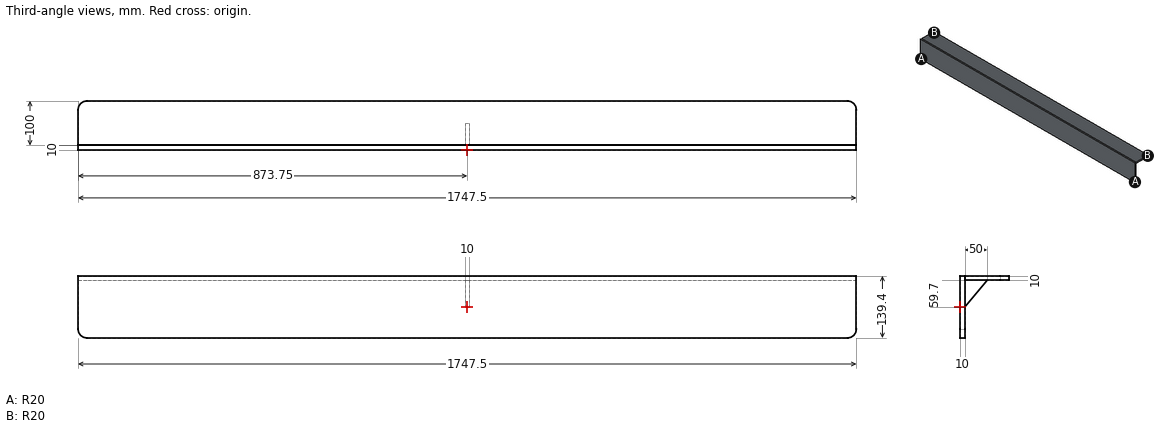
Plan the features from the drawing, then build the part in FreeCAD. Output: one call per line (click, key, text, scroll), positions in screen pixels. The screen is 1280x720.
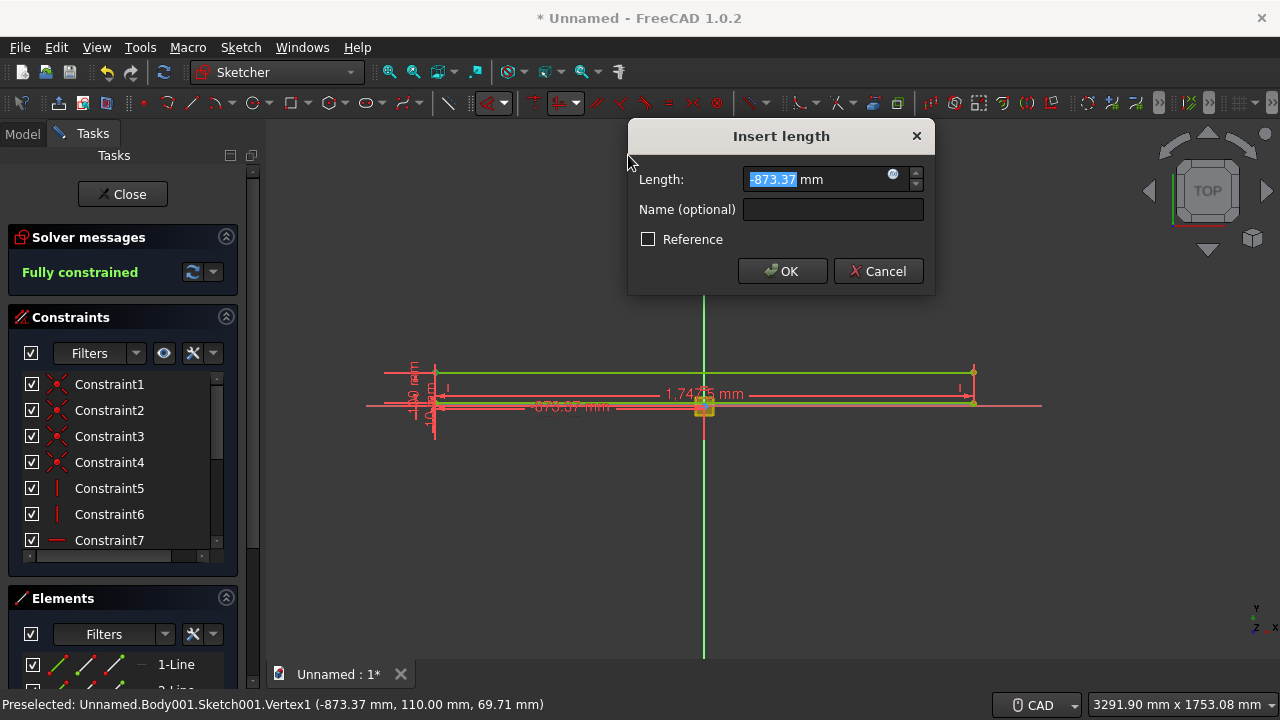
text(-873.75)
key(Return)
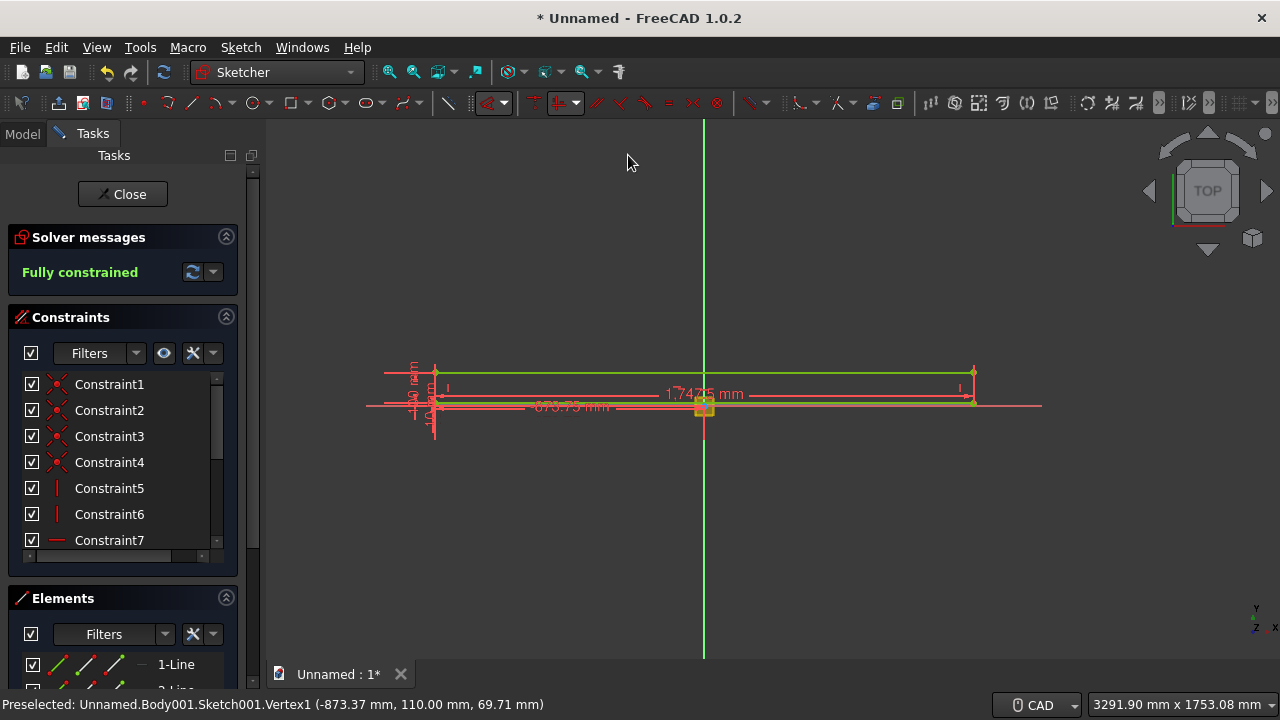
click(123, 194)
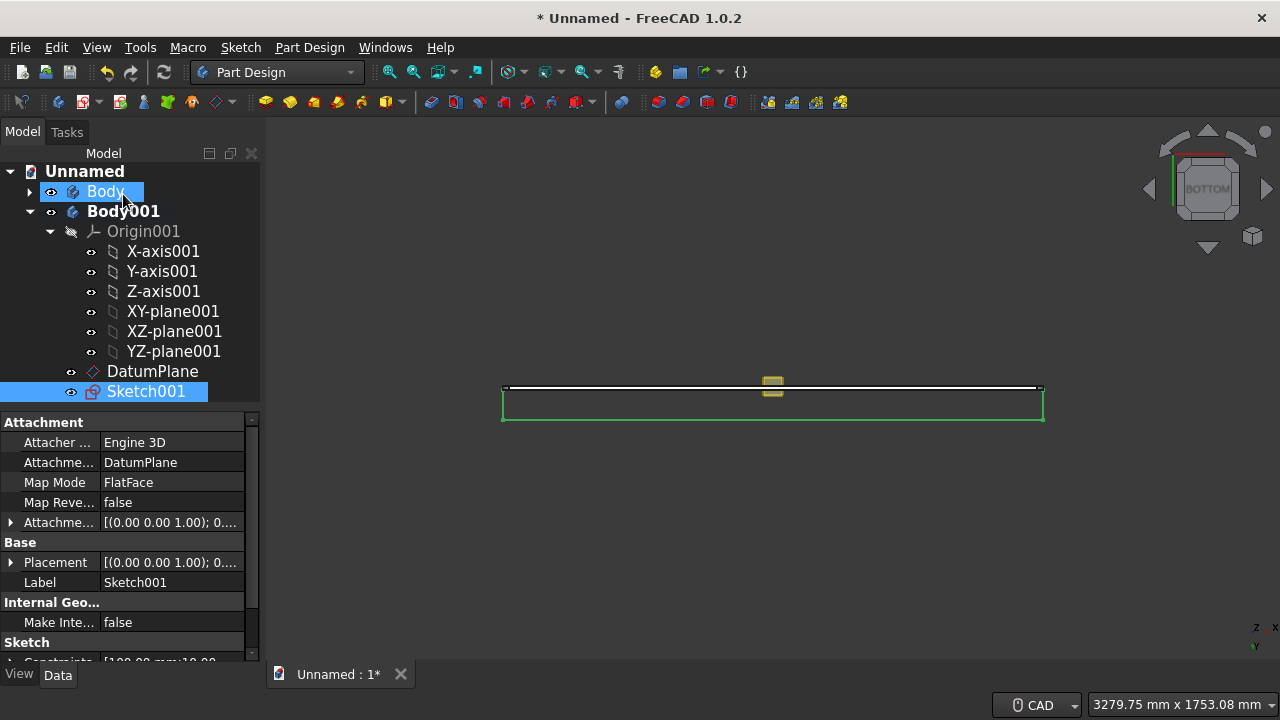
click(266, 102)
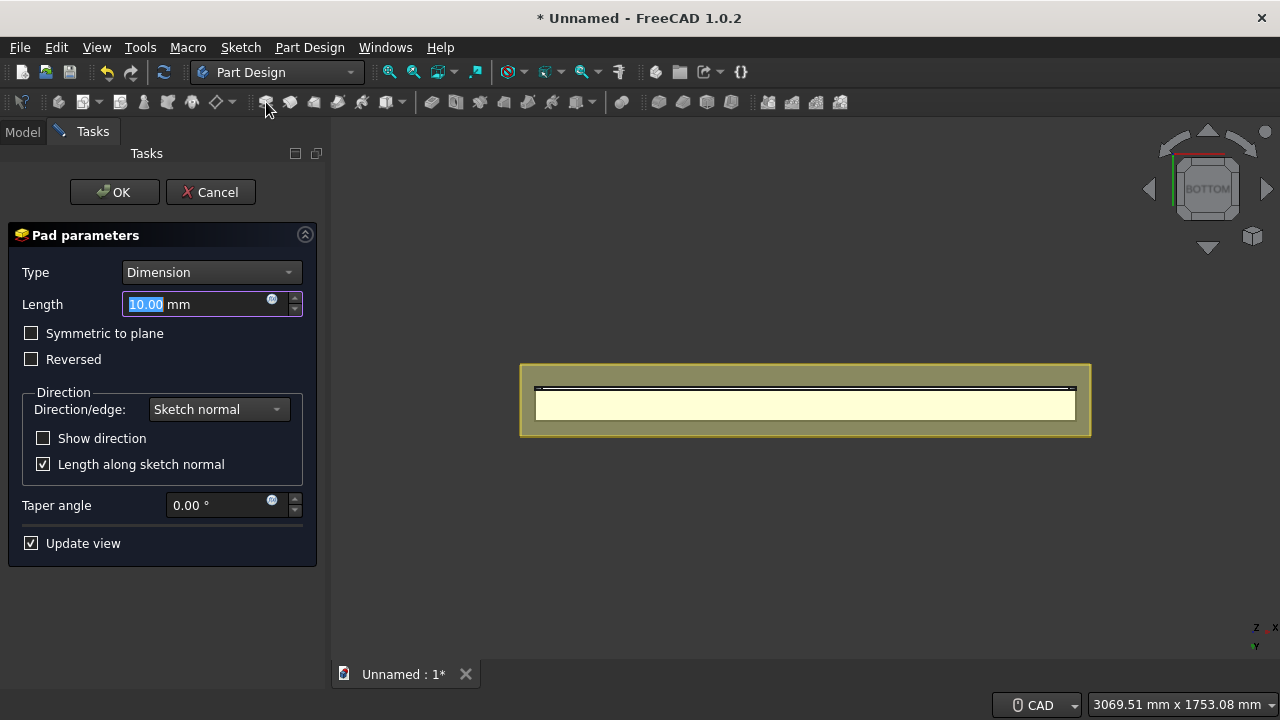
text(10)
key(Tab)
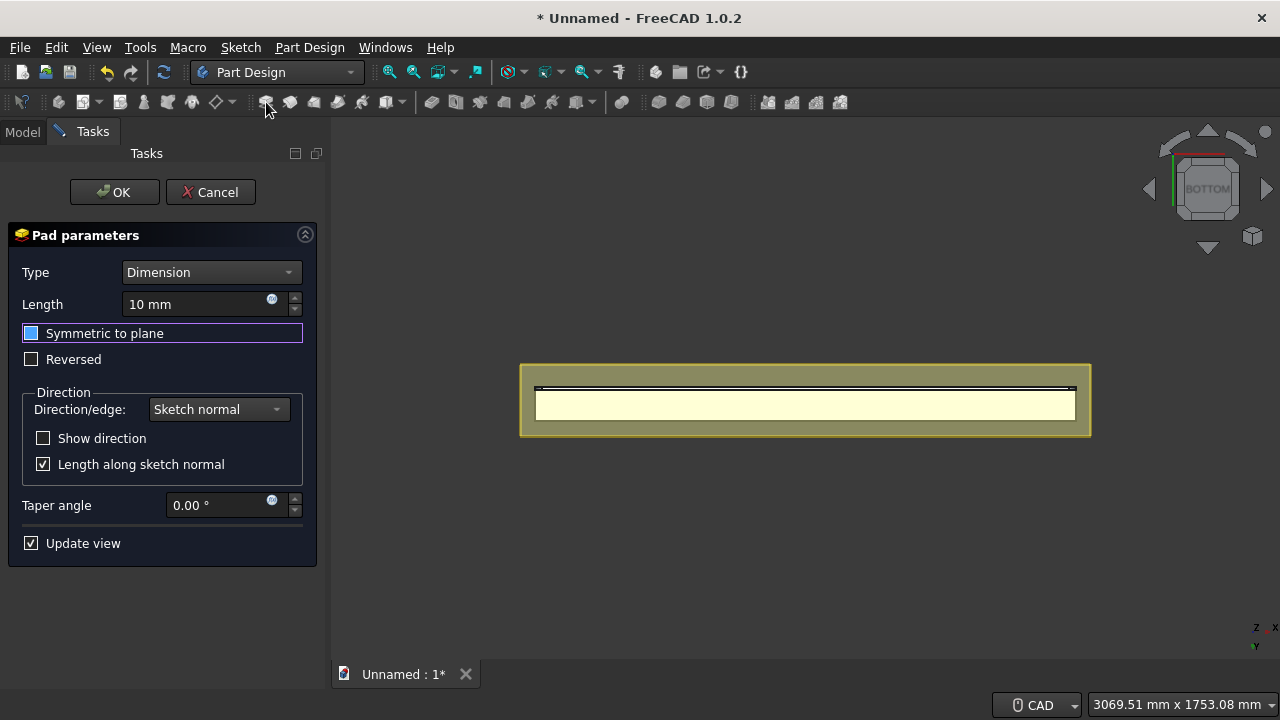
click(30, 359)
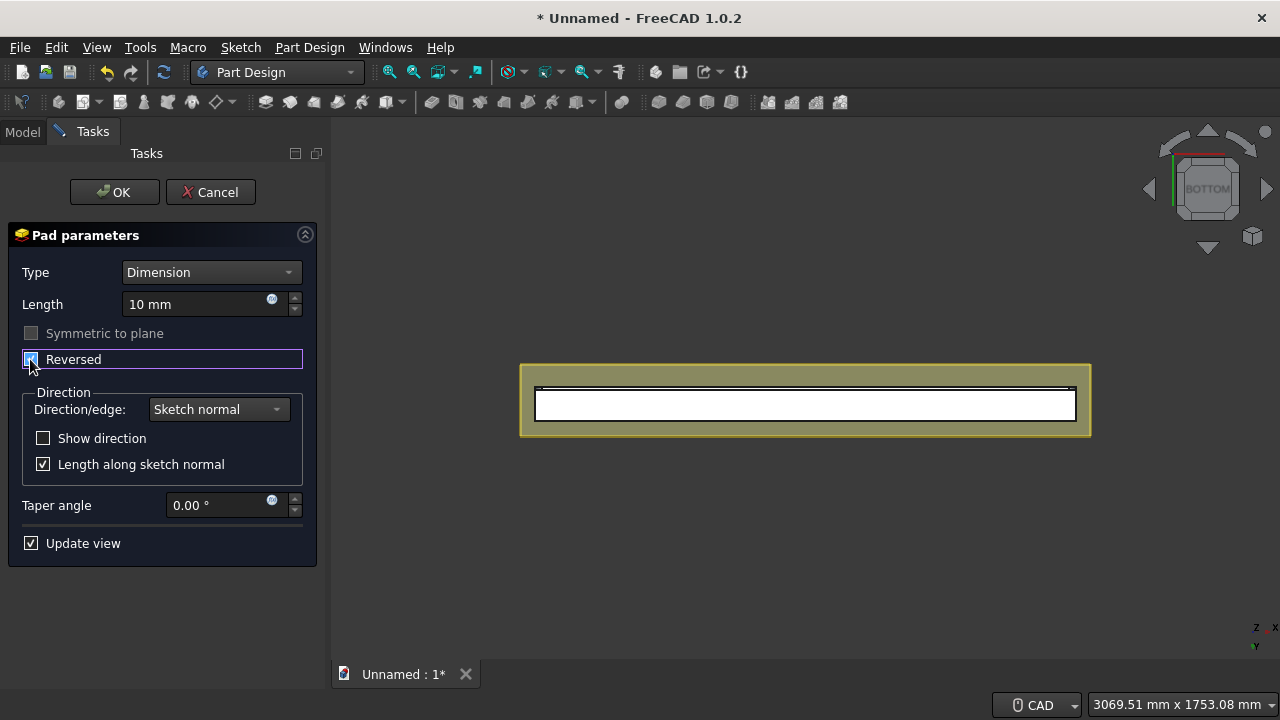
click(115, 192)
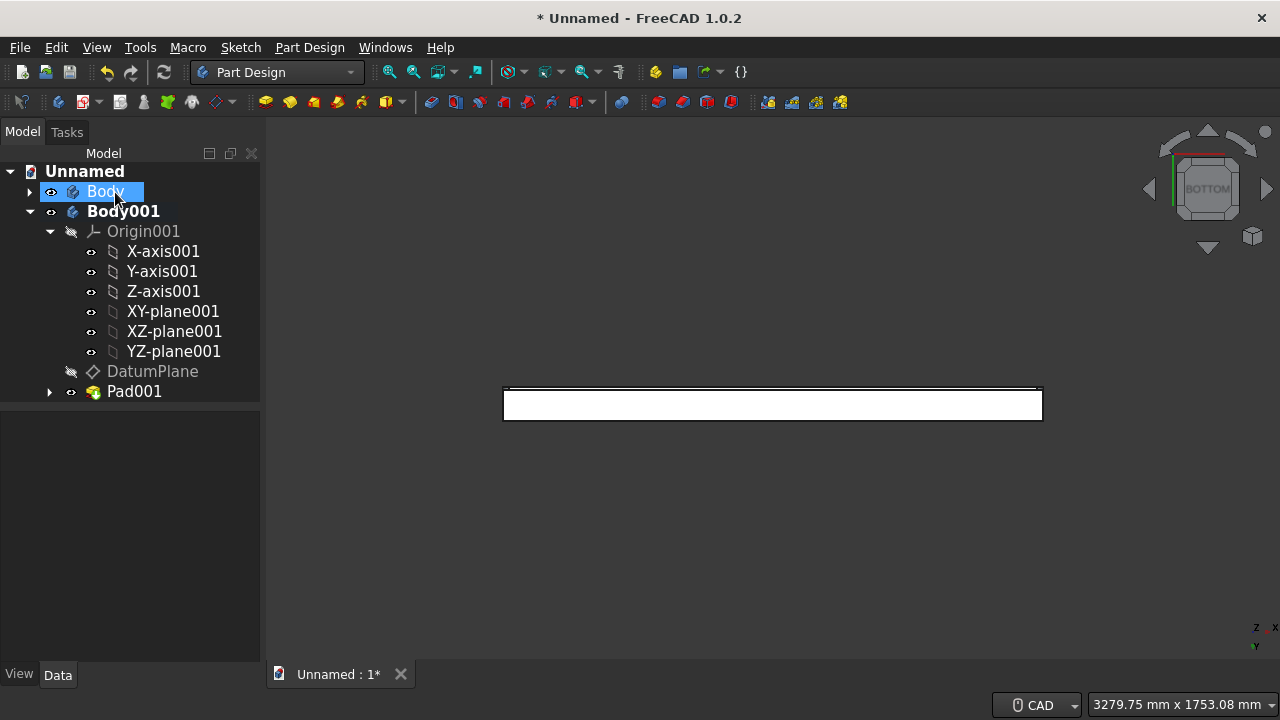
scroll(503, 420, up, 13)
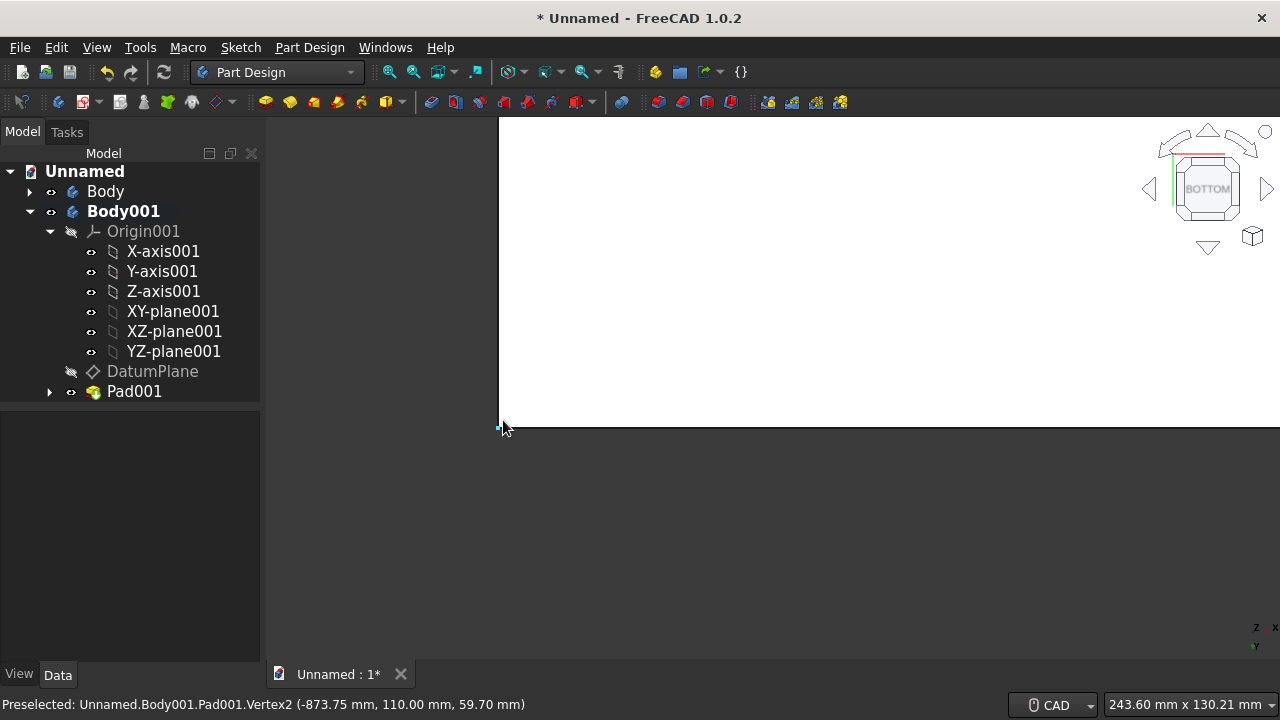
click(390, 72)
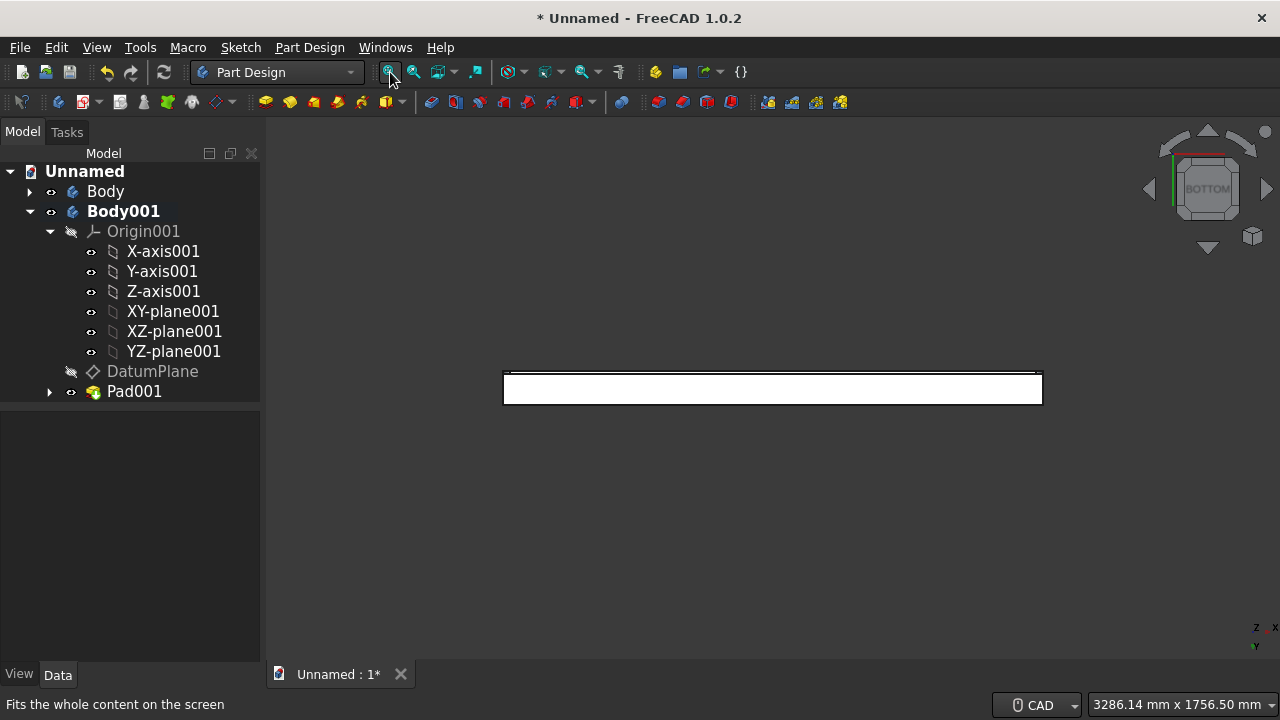
key(0)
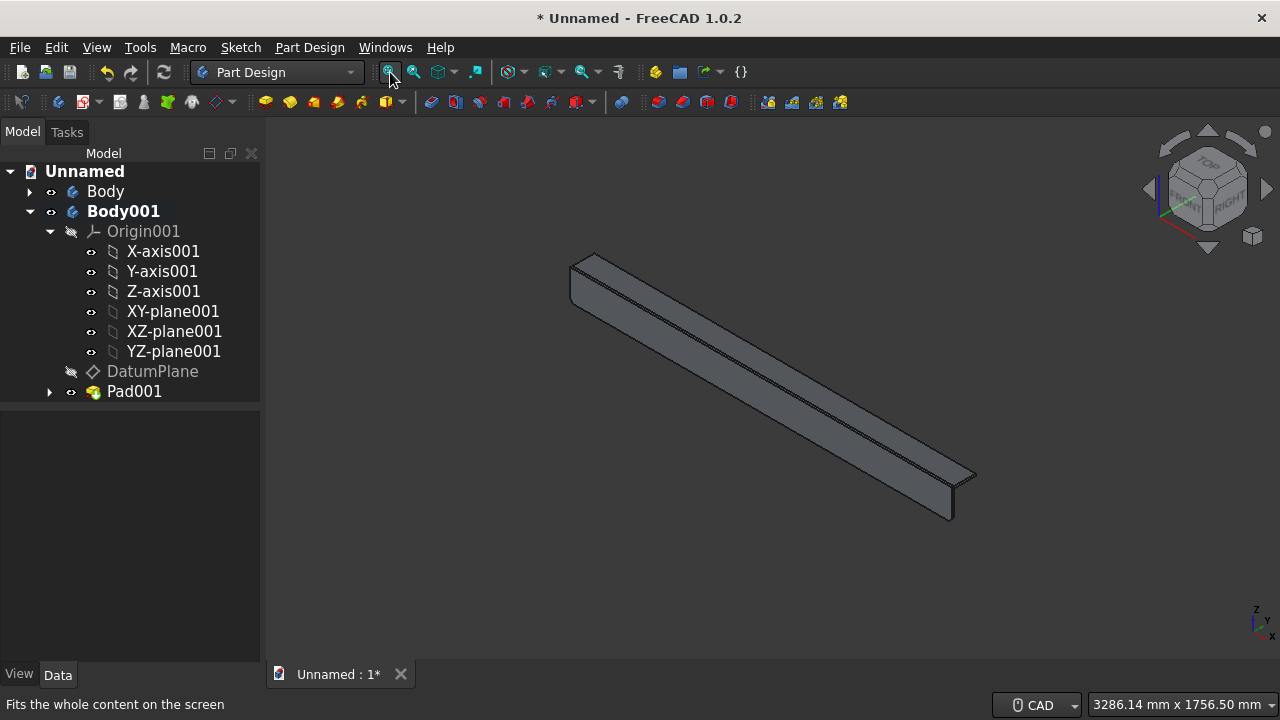
click(390, 72)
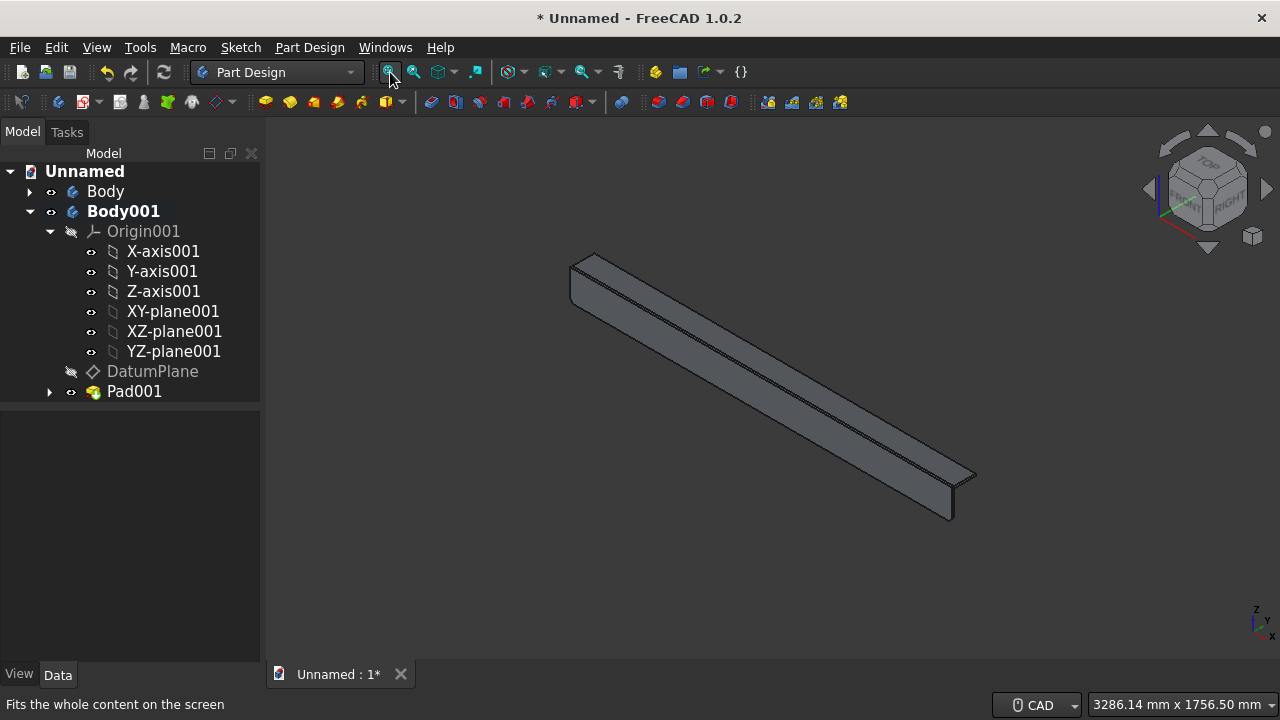
scroll(594, 254, up, 13)